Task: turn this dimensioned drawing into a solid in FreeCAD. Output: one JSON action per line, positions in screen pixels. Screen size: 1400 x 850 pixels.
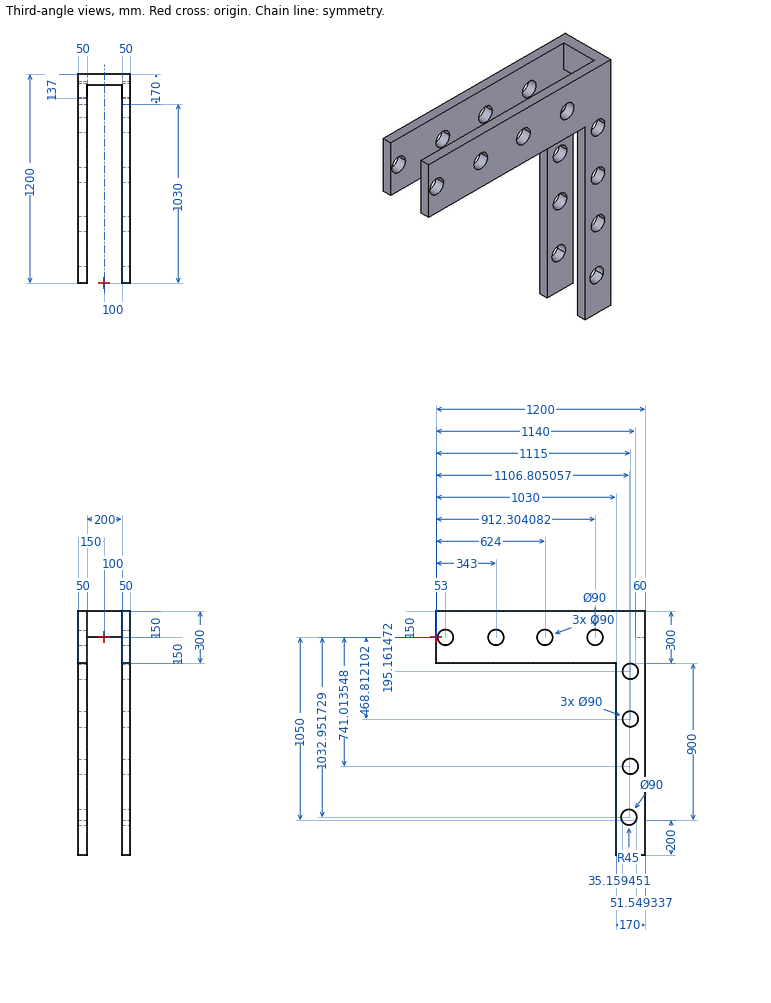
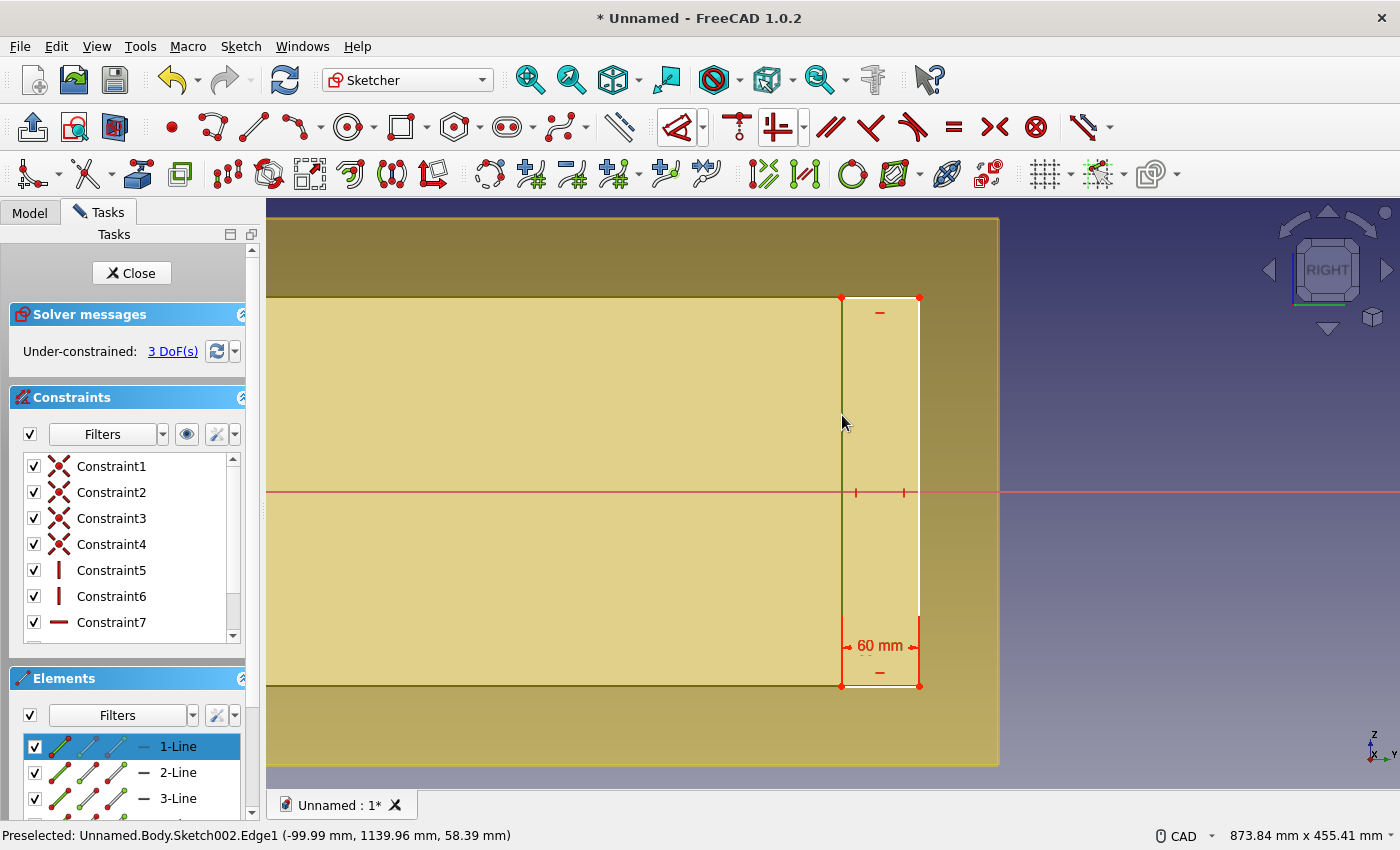
{"action": "left_click", "coordinate": [702, 128]}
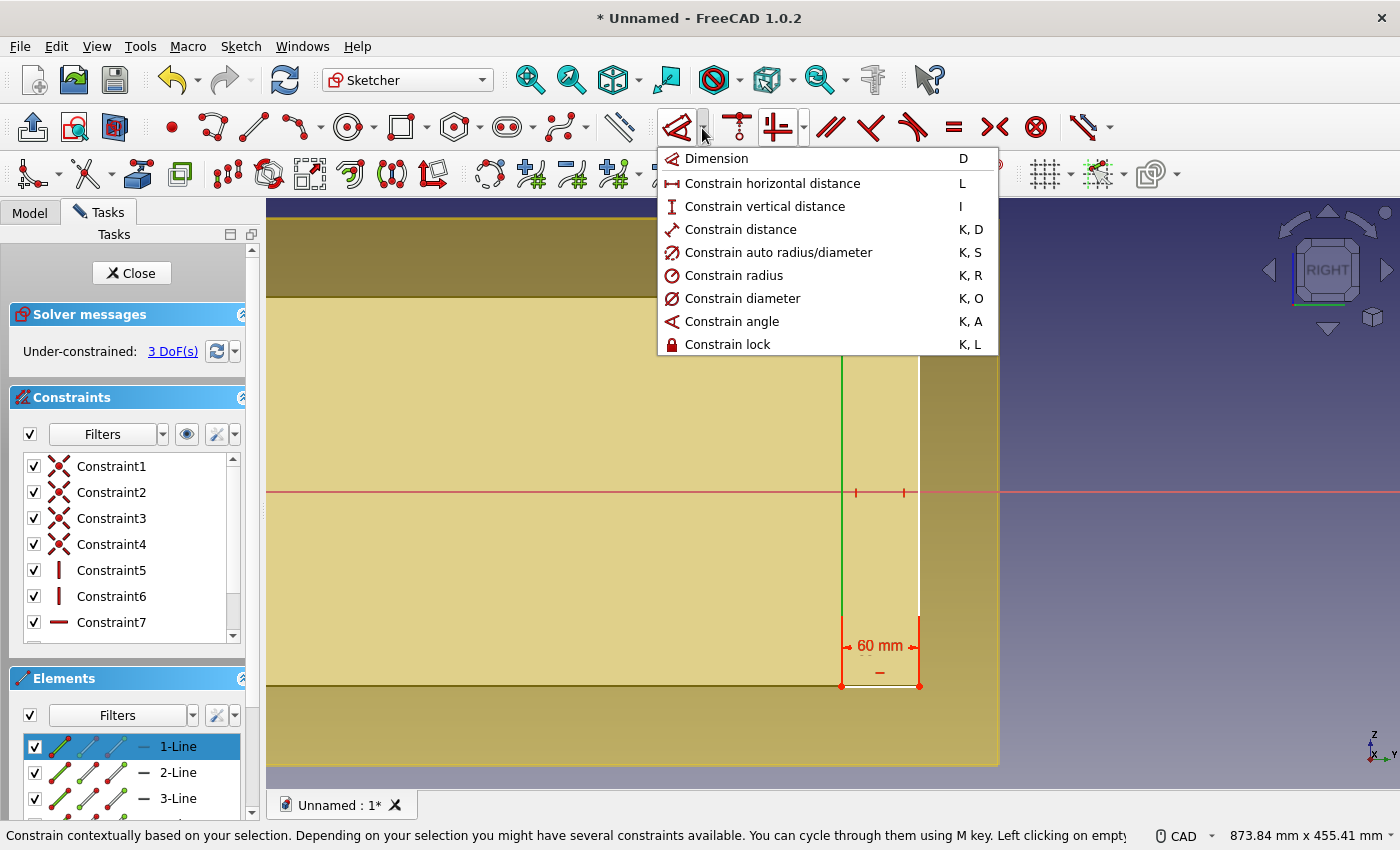
{"action": "left_click", "coordinate": [828, 206]}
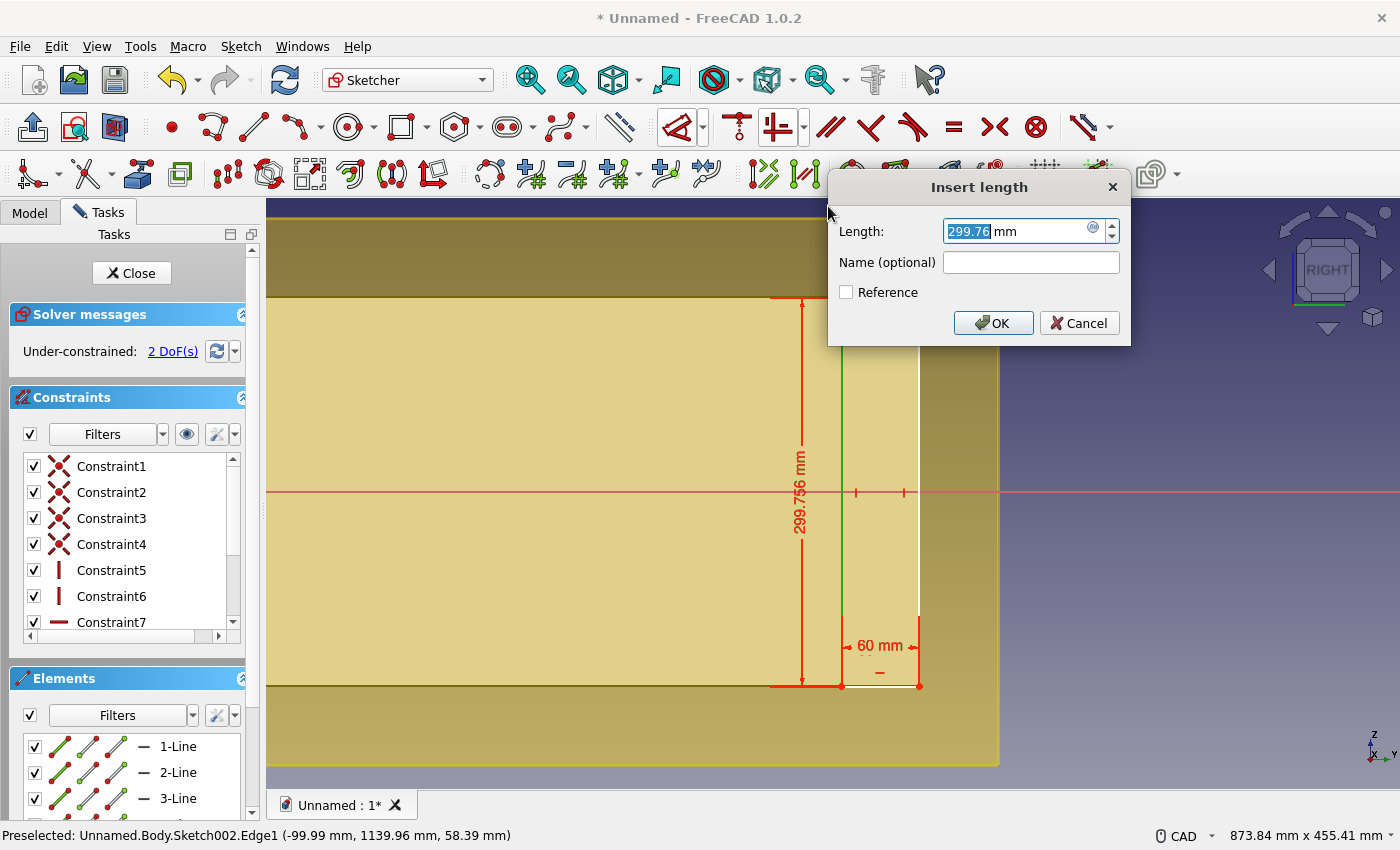
{"action": "type", "text": "300"}
{"action": "key", "text": "Return"}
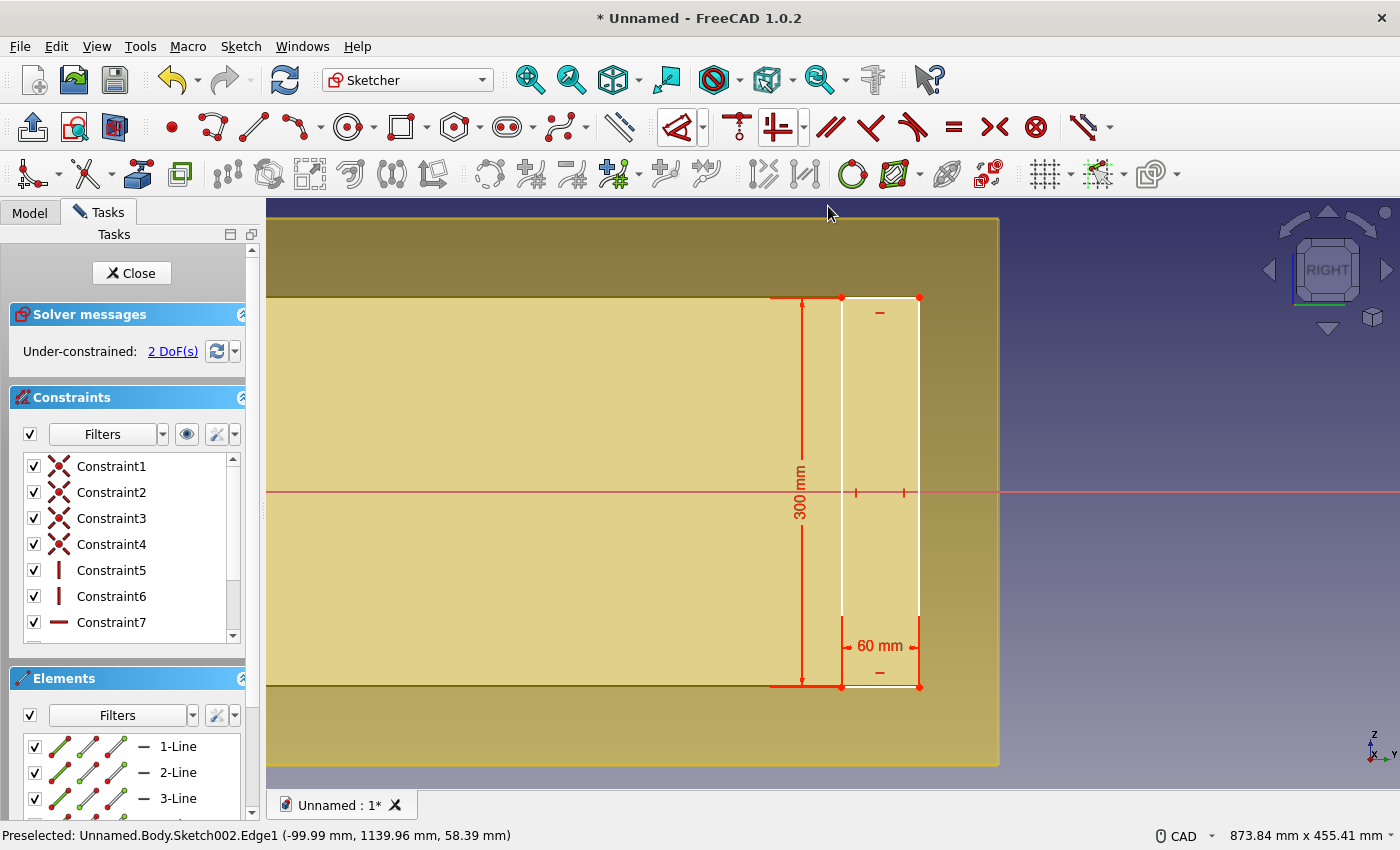
{"action": "left_click", "coordinate": [842, 298]}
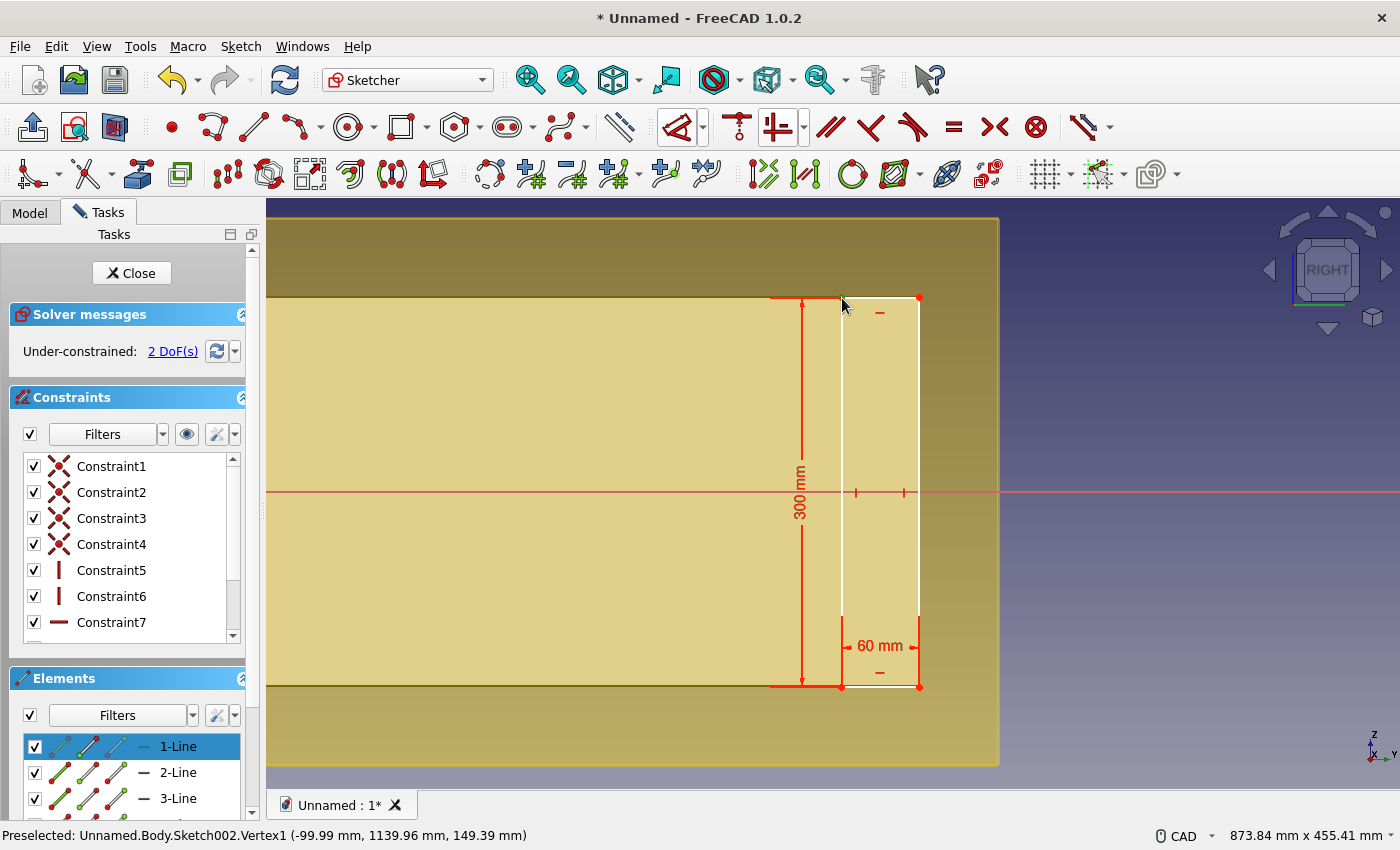
{"action": "left_click", "coordinate": [702, 128]}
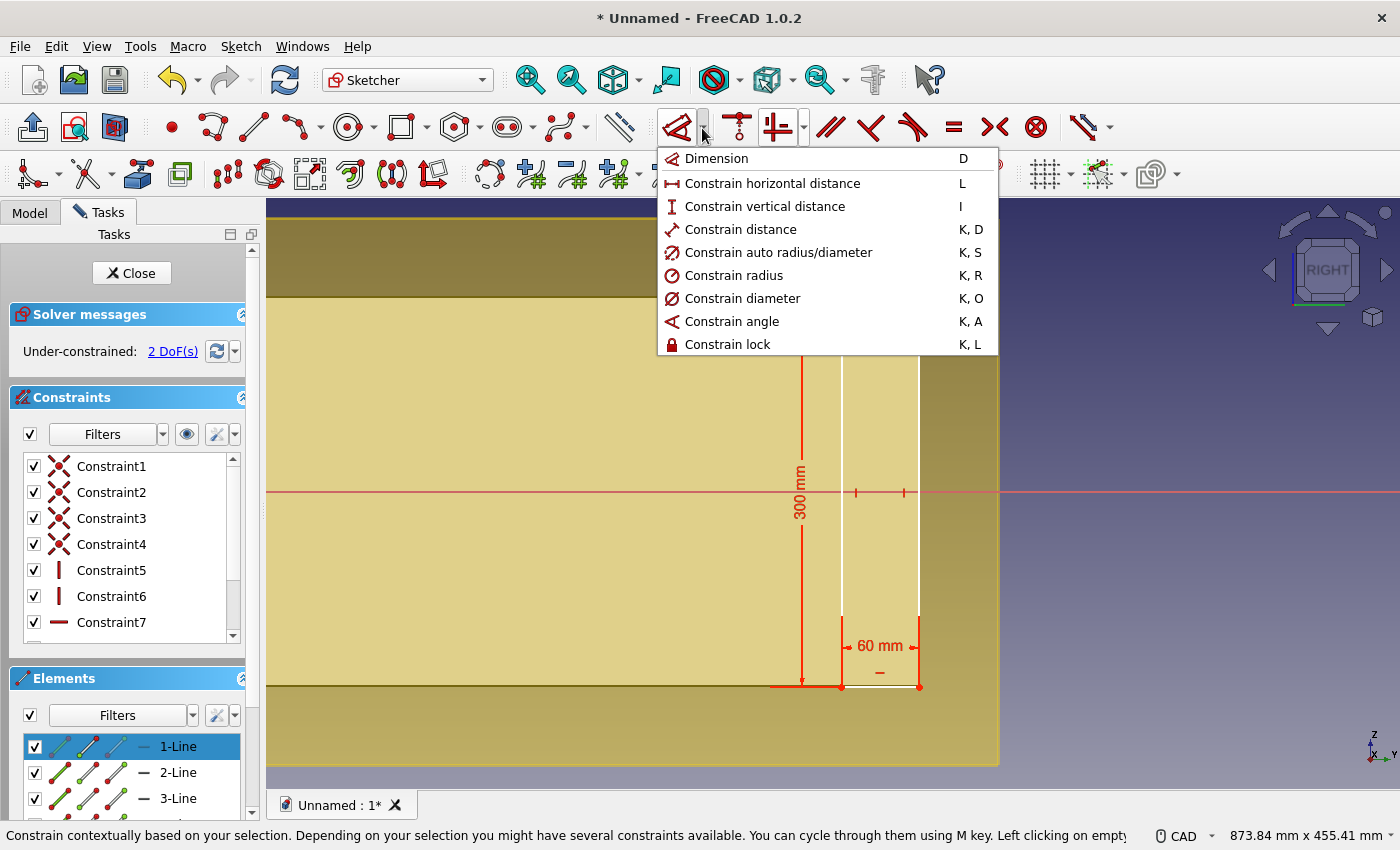
{"action": "left_click", "coordinate": [828, 206]}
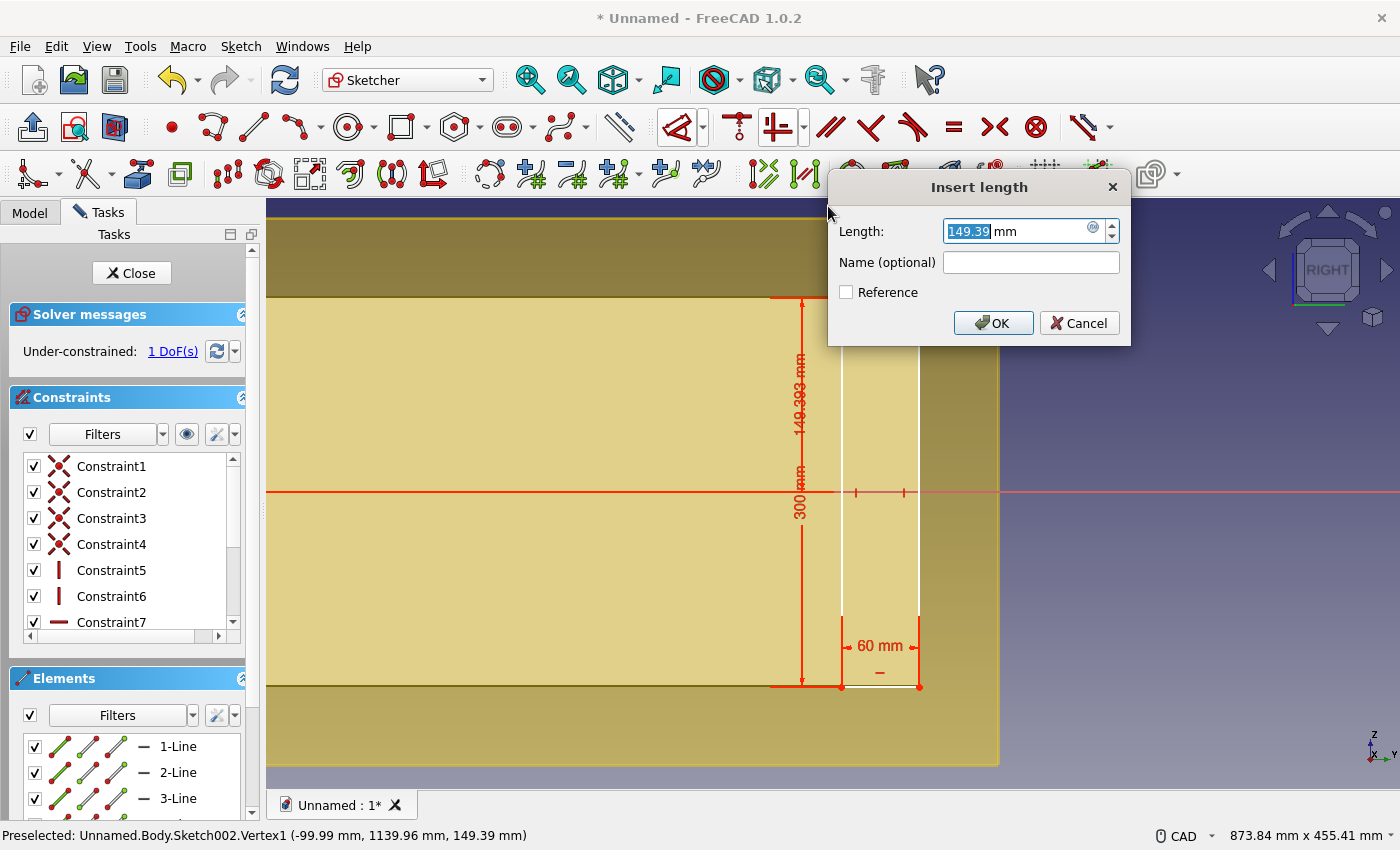
{"action": "type", "text": "150"}
{"action": "key", "text": "Return"}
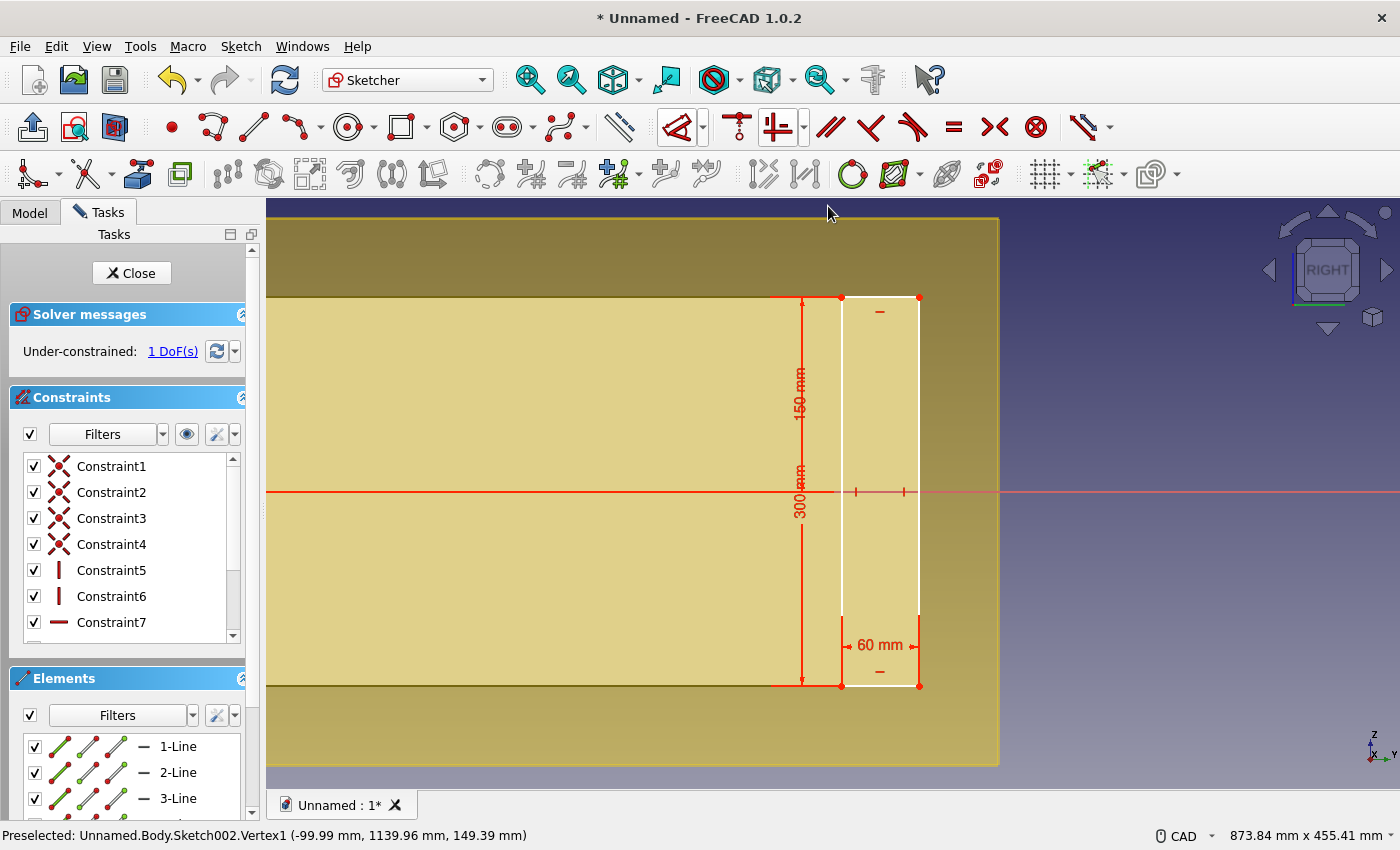
{"action": "left_click", "coordinate": [842, 297]}